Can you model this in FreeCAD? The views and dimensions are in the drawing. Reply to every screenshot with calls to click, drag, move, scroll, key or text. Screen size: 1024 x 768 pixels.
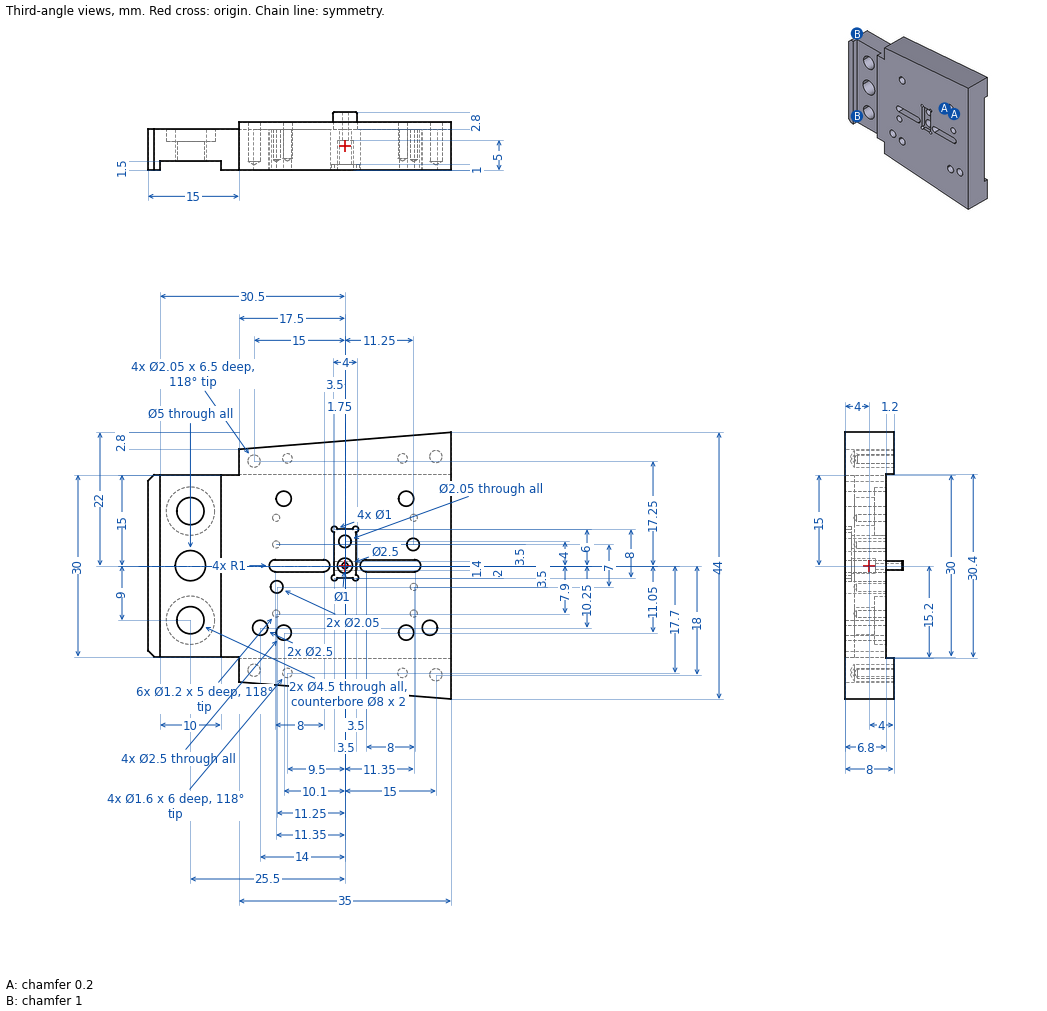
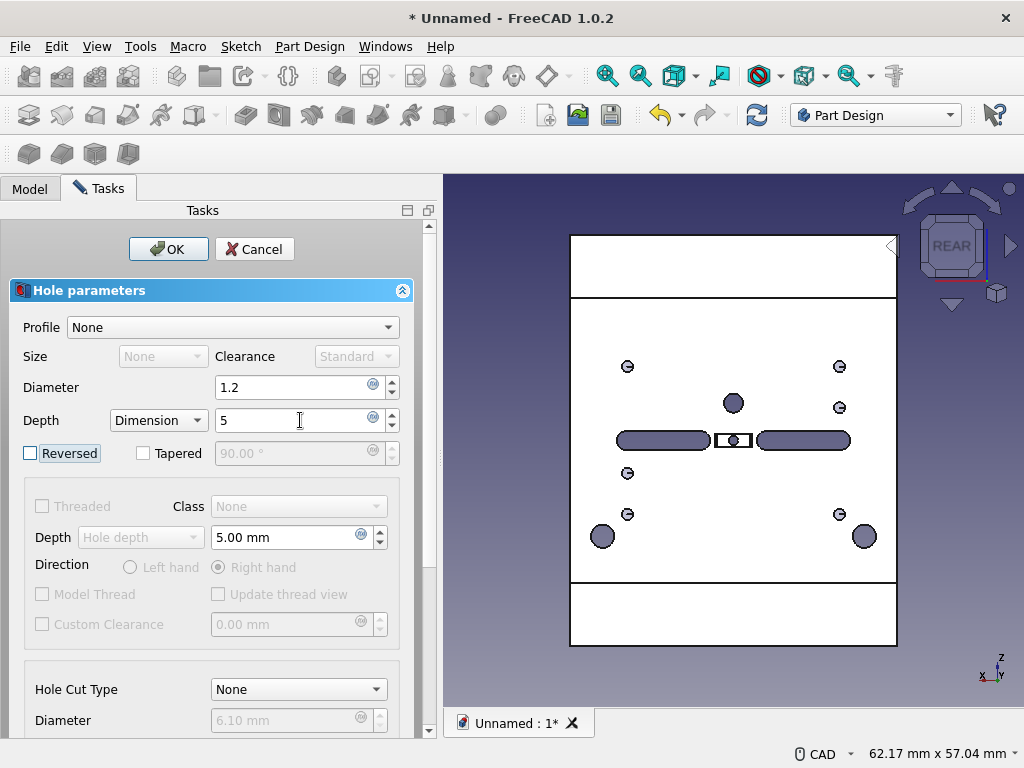
click(169, 249)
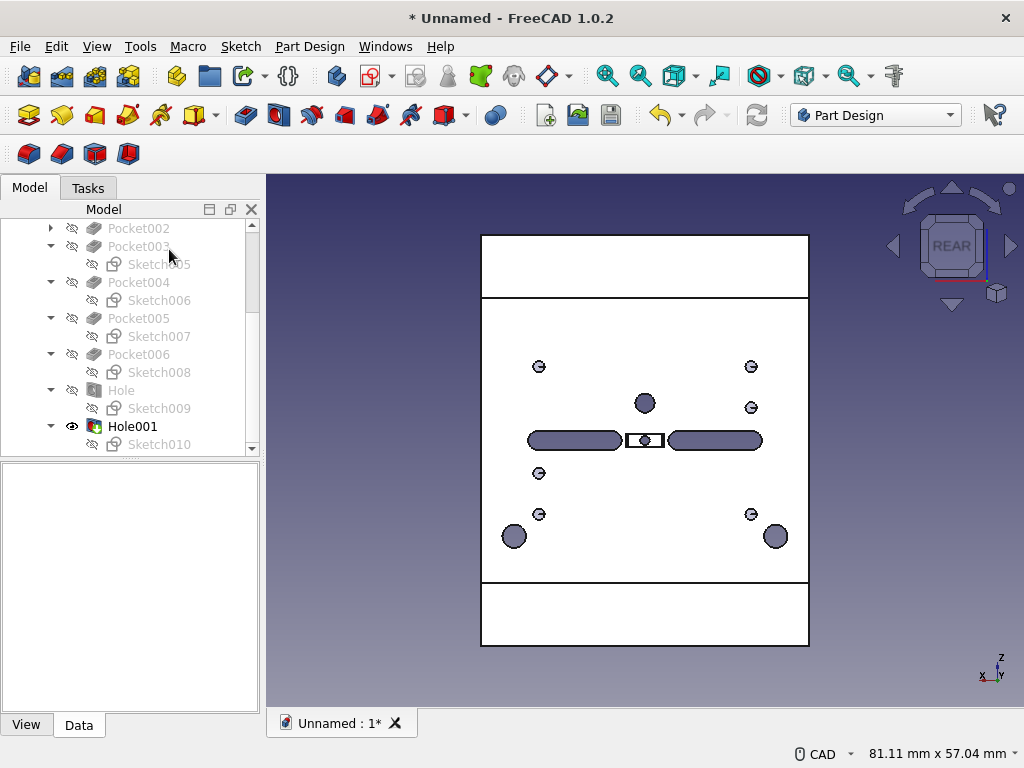
click(645, 521)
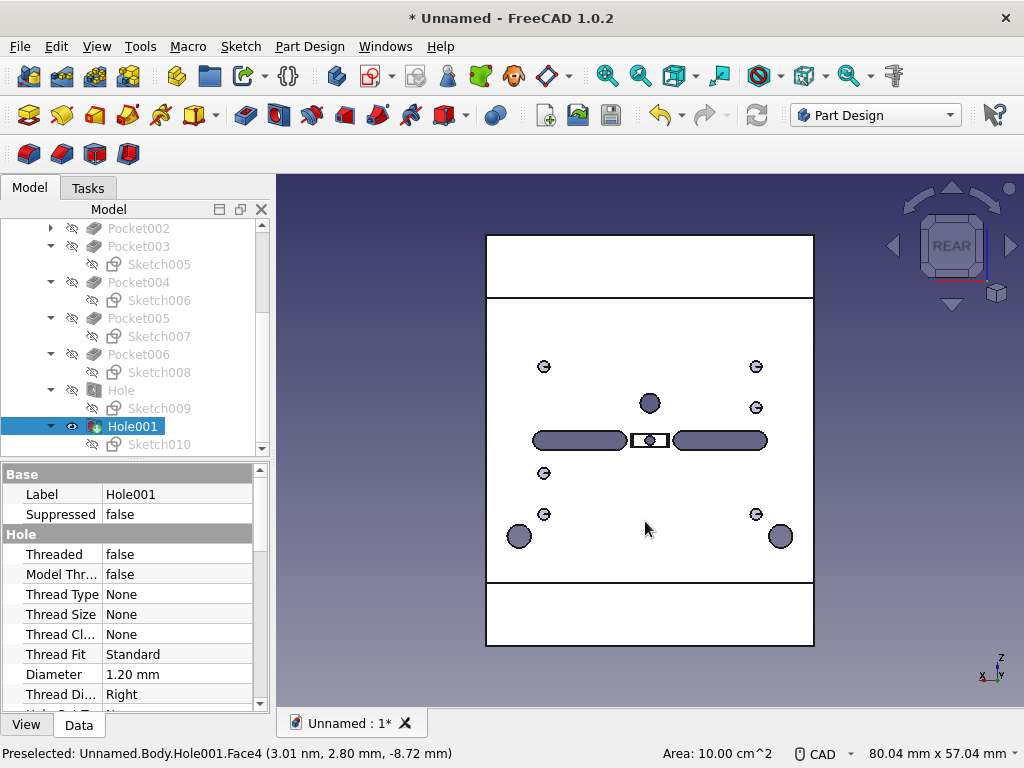
click(370, 76)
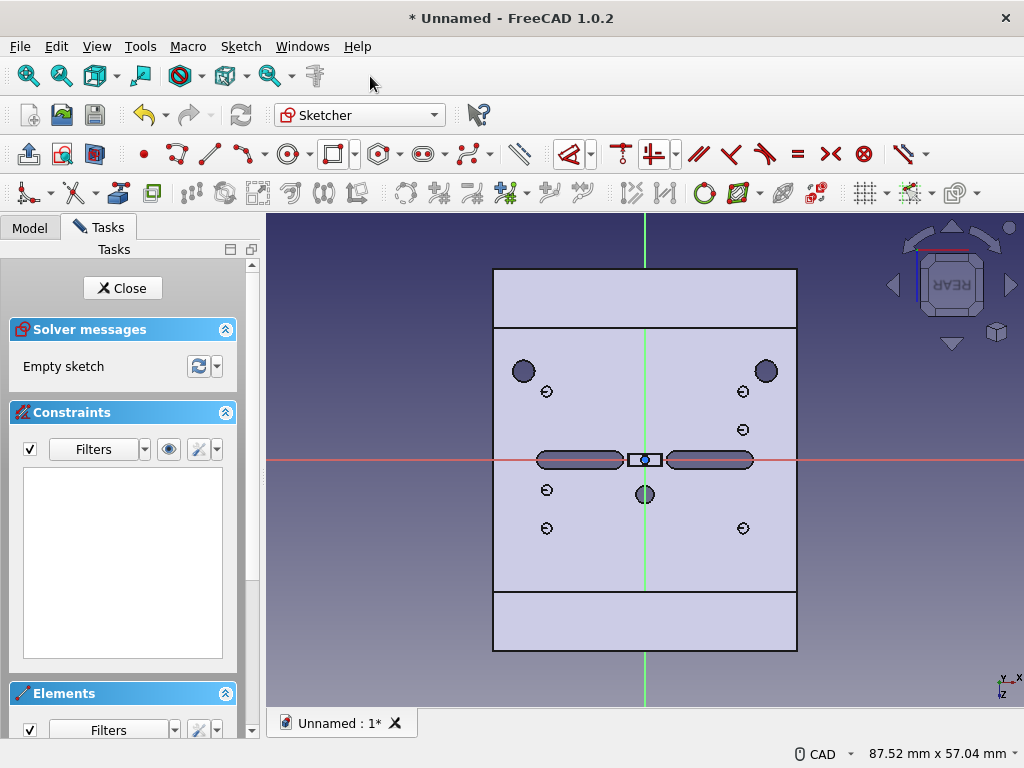
click(95, 154)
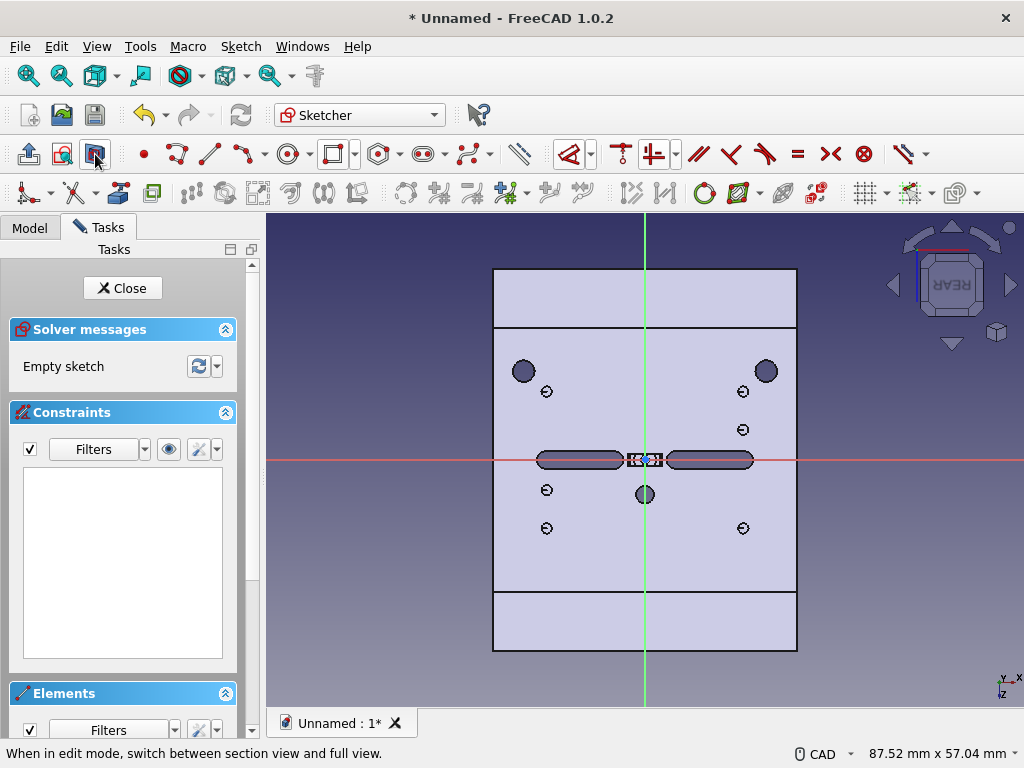
scroll(728, 460, up, 3)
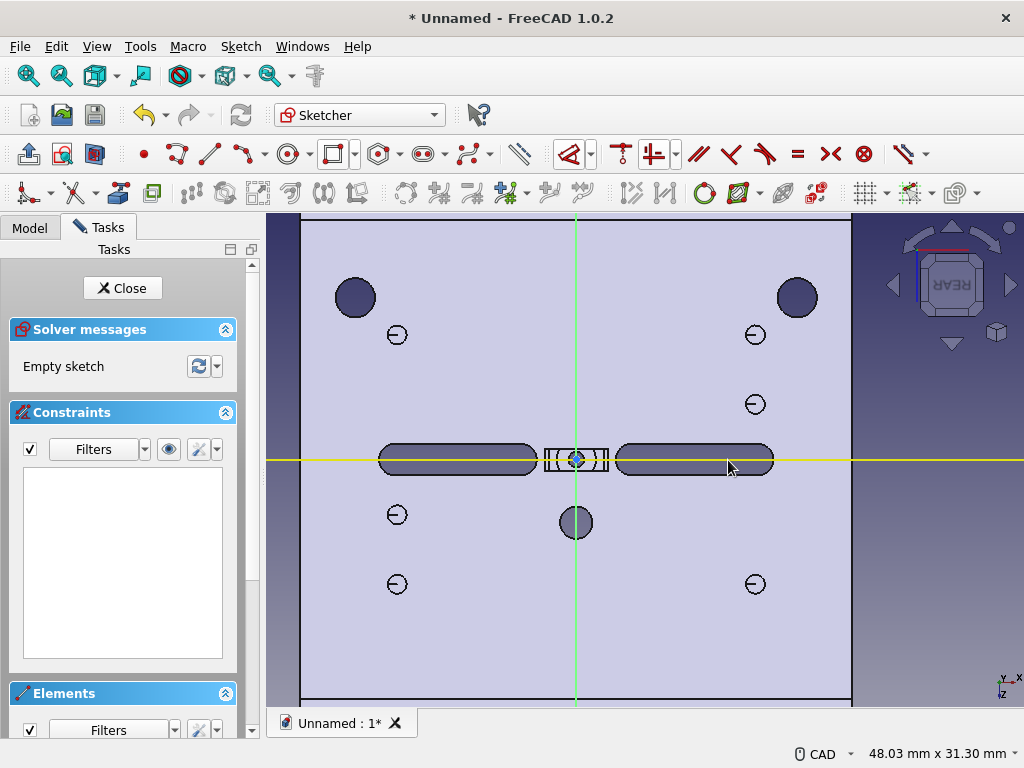
click(288, 154)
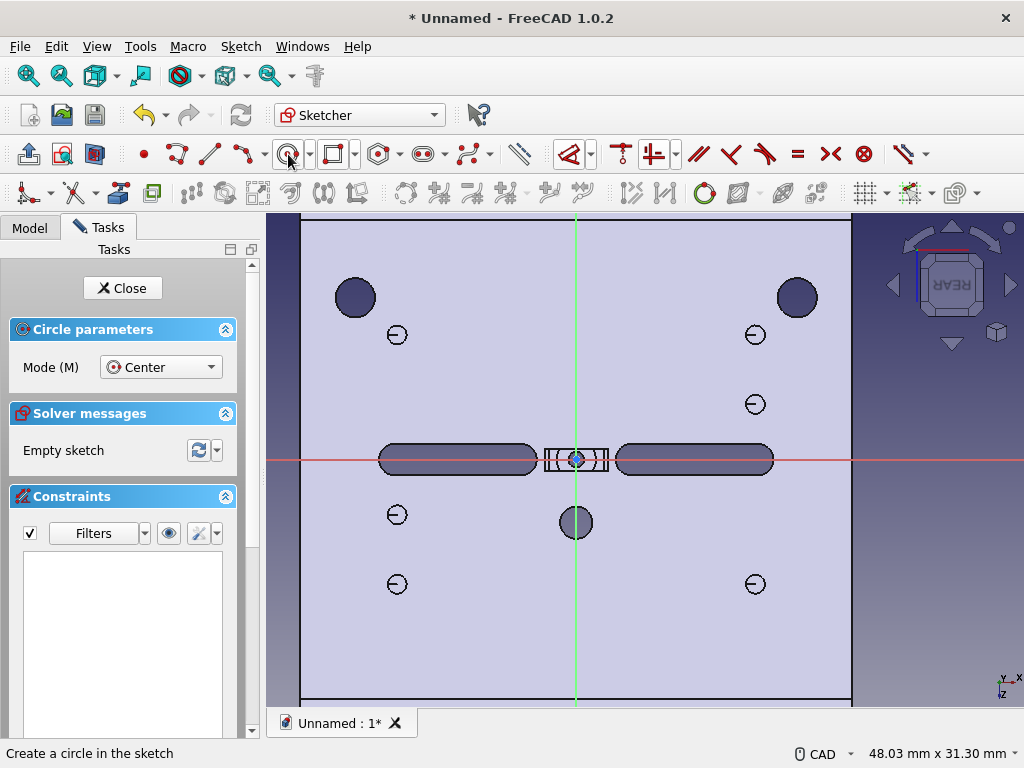
scroll(399, 404, up, 2)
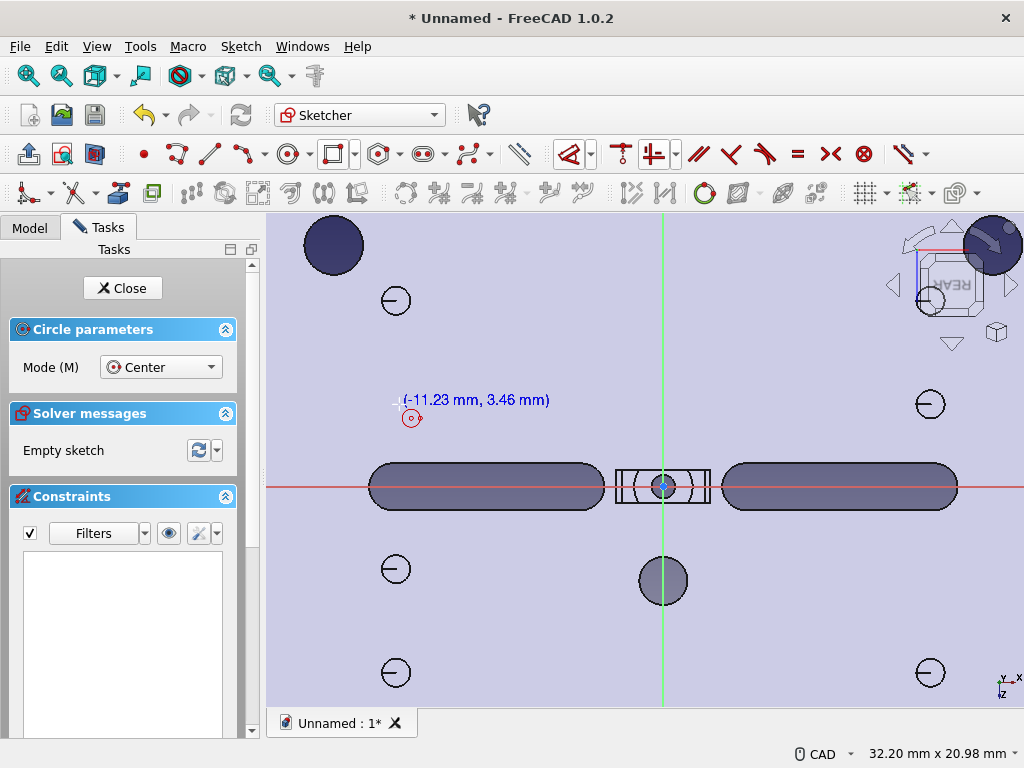
click(398, 404)
move(416, 387)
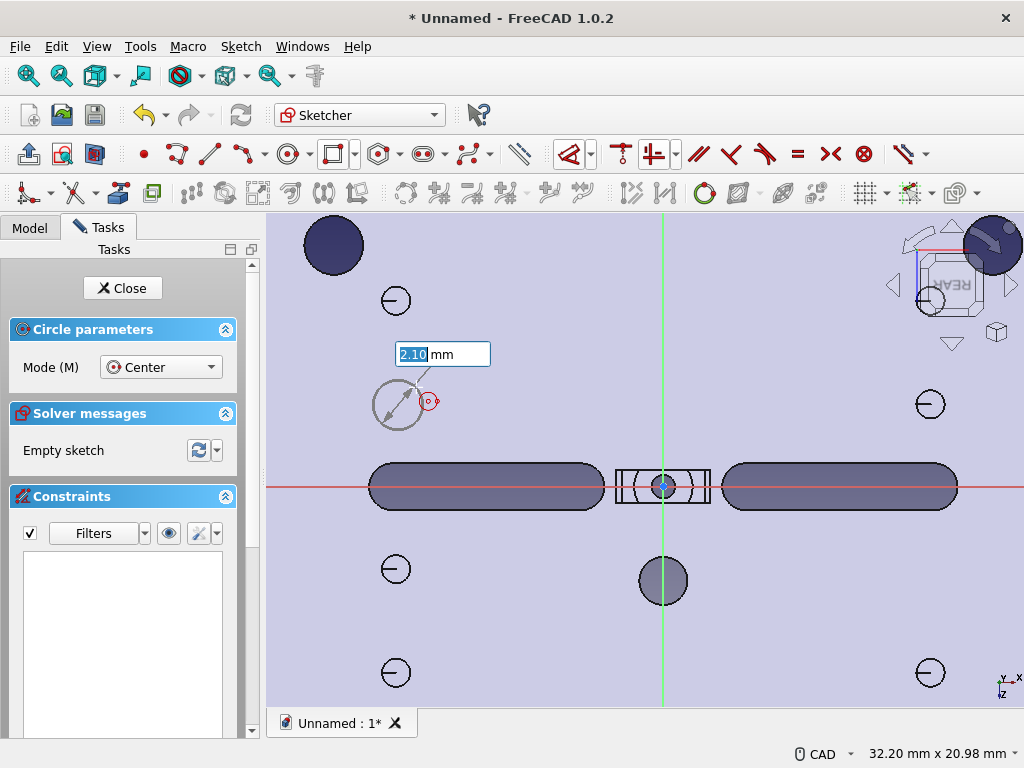
text(2.05)
key(Return)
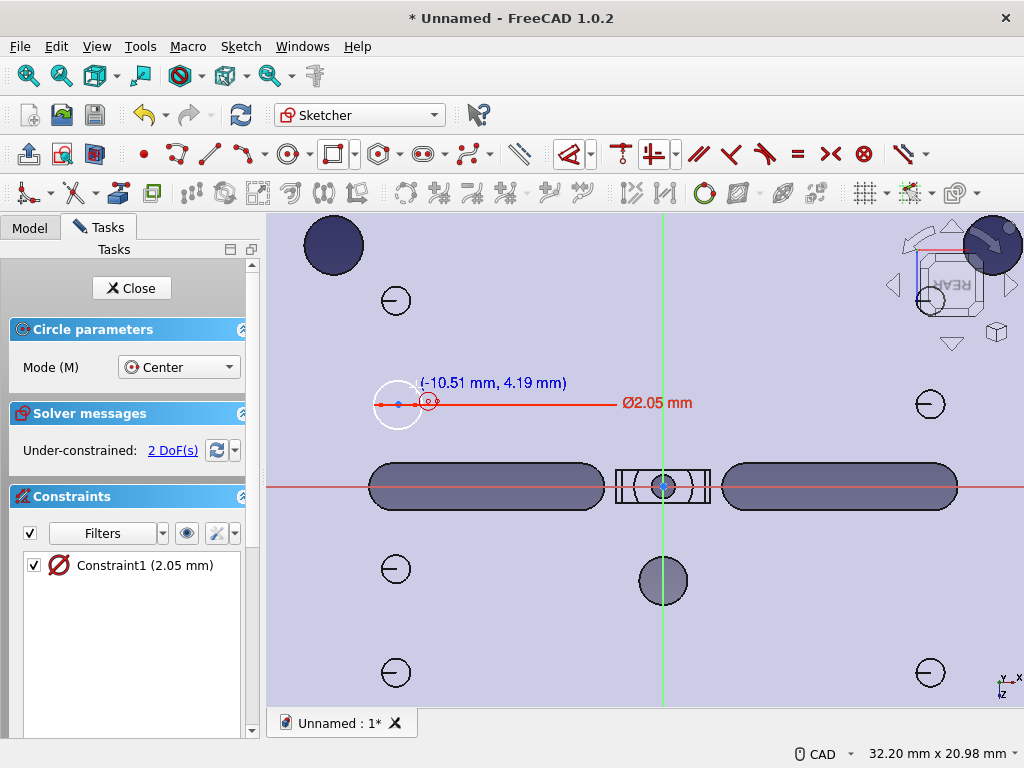
scroll(400, 406, down, 2)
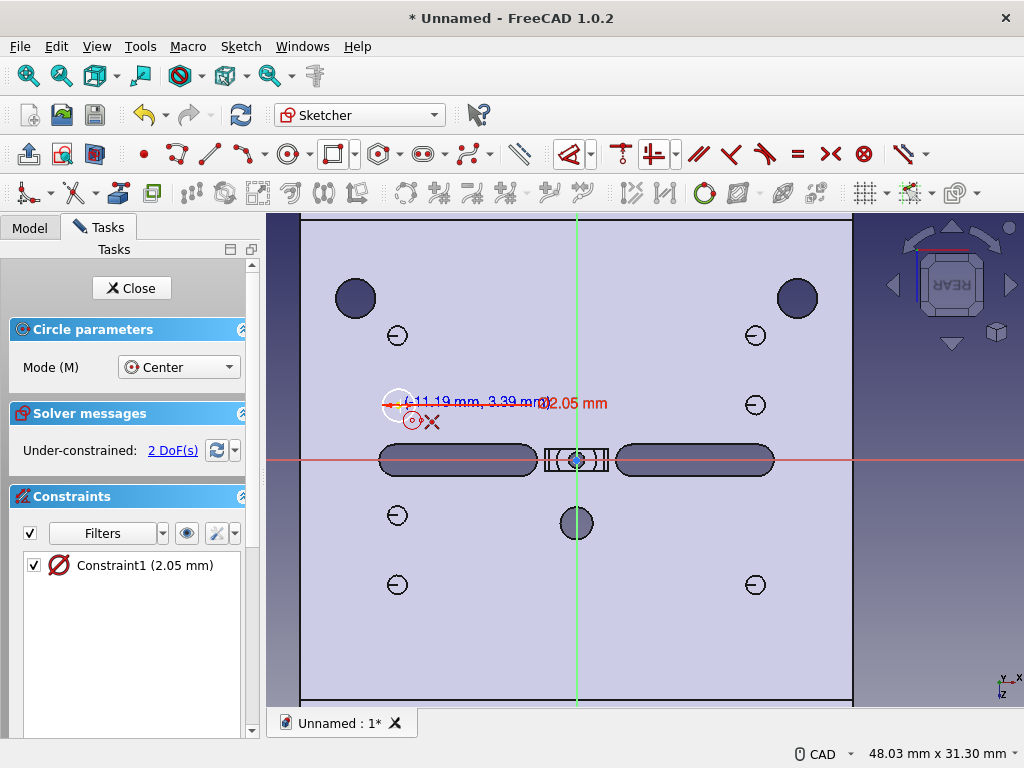
scroll(754, 515, up, 2)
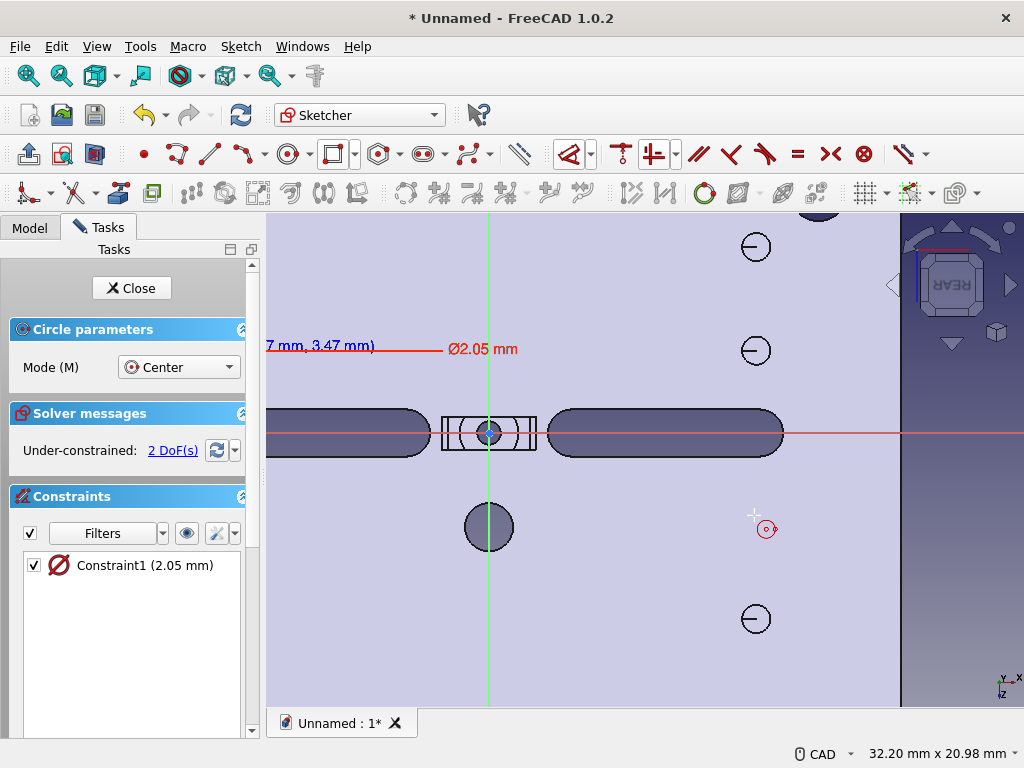
click(754, 515)
move(771, 498)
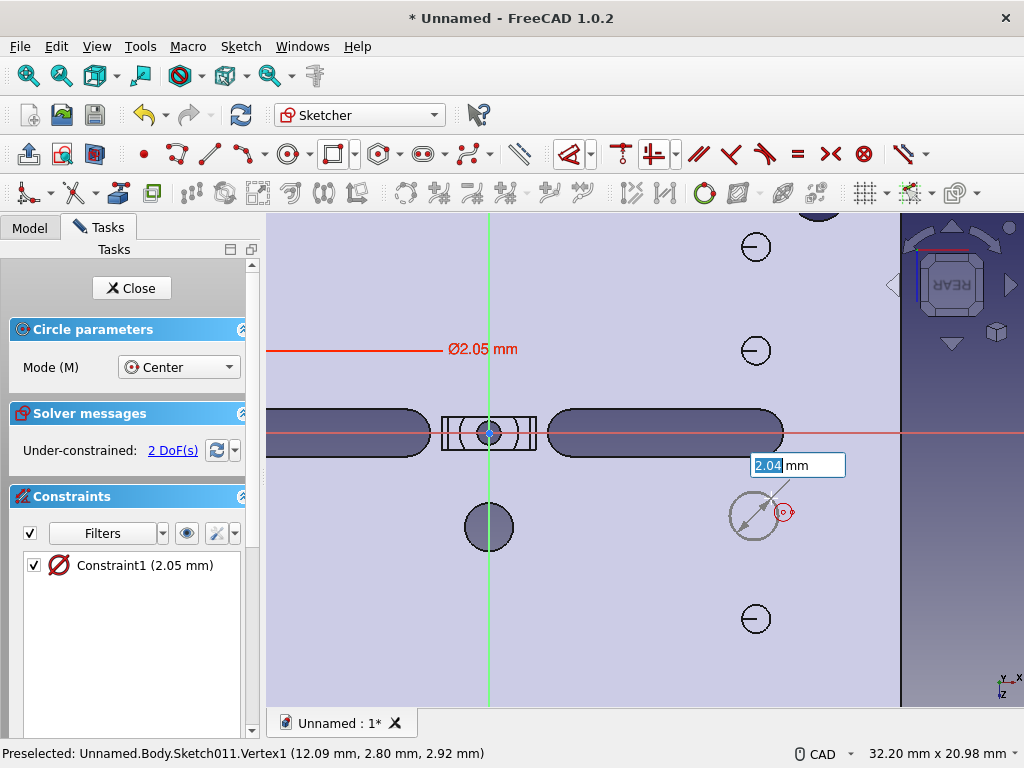
text(2.05)
key(Return)
key(Escape)